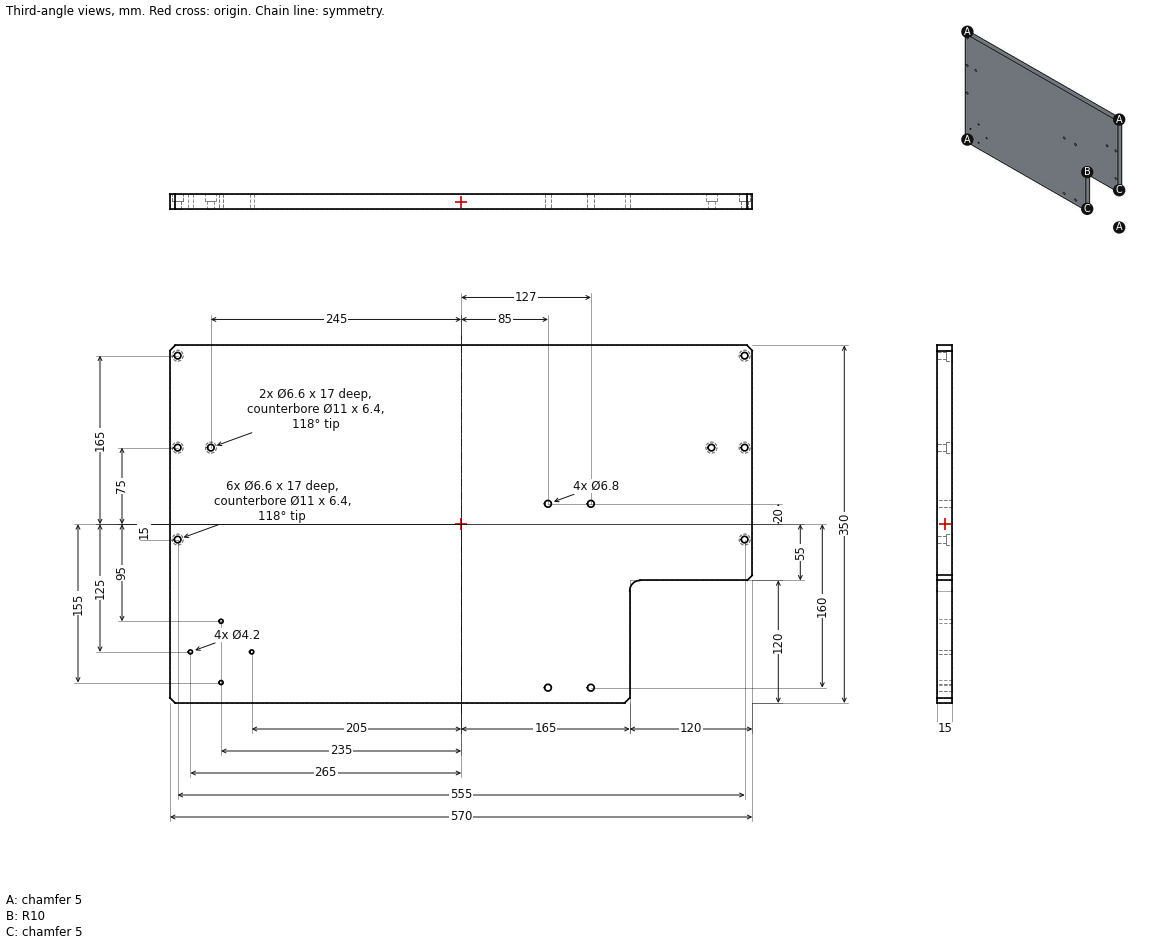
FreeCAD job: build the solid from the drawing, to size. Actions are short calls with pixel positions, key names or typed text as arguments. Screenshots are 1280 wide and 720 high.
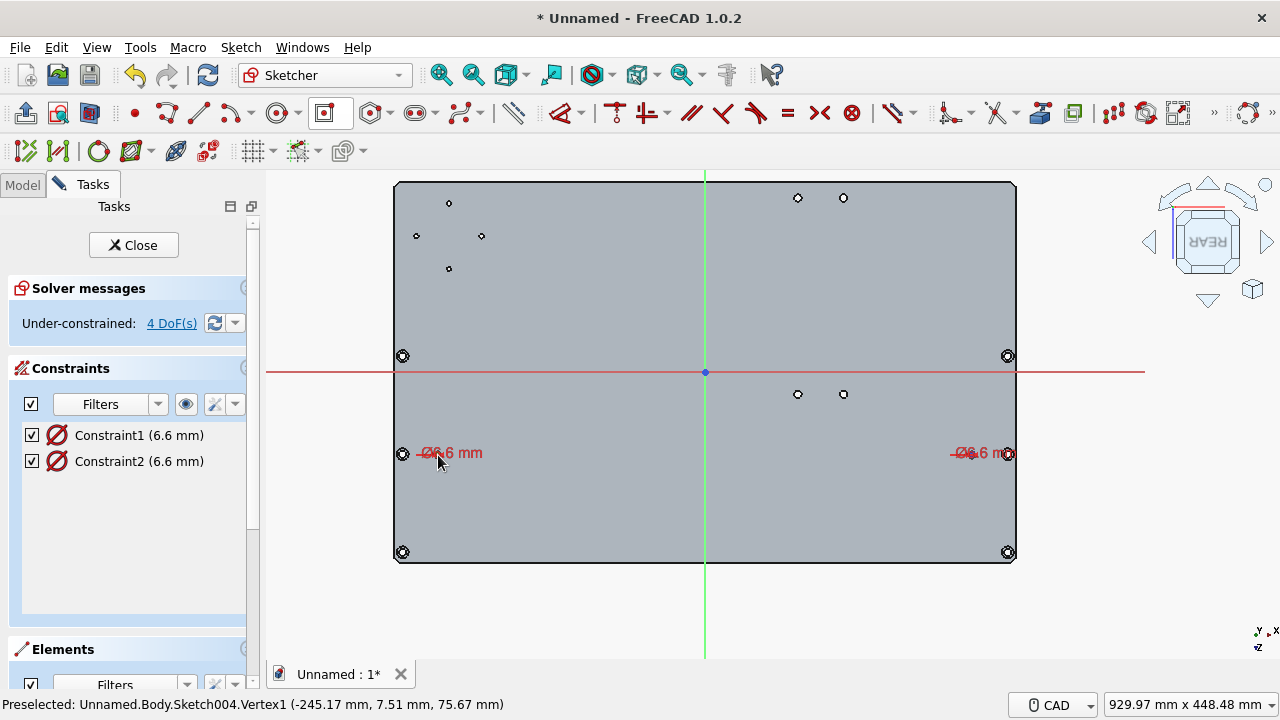
click(972, 455)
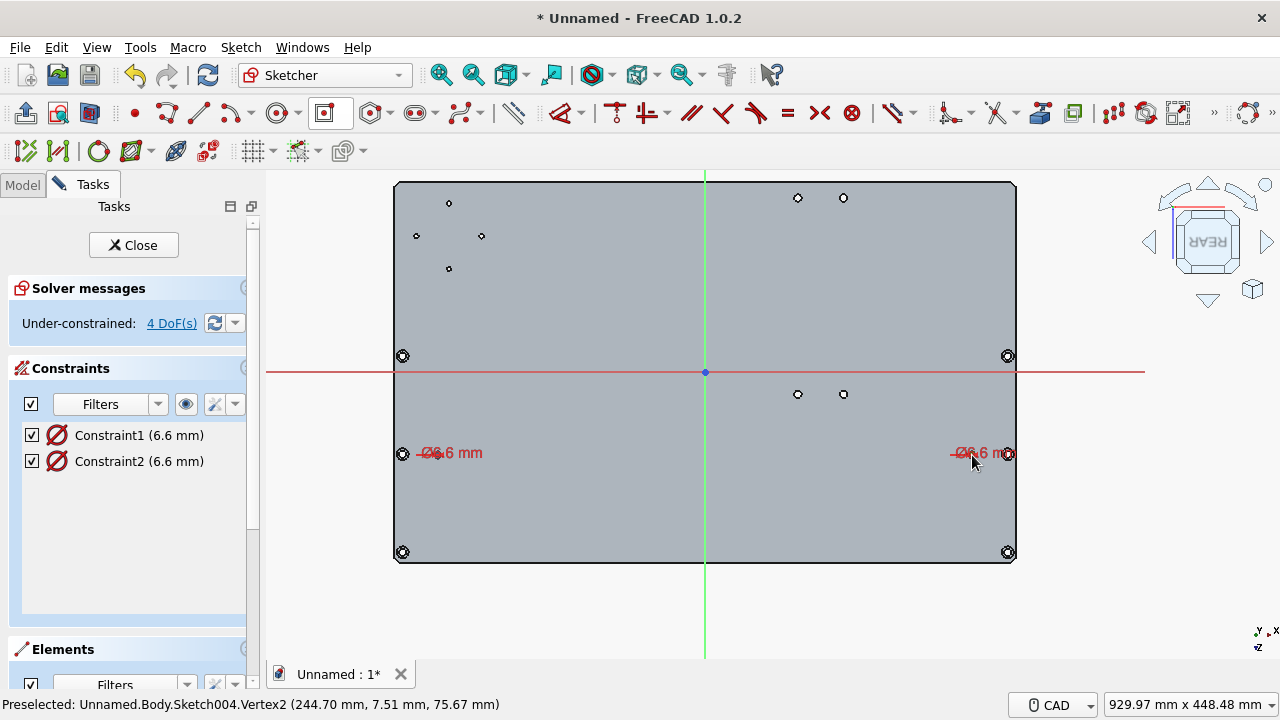
click(705, 600)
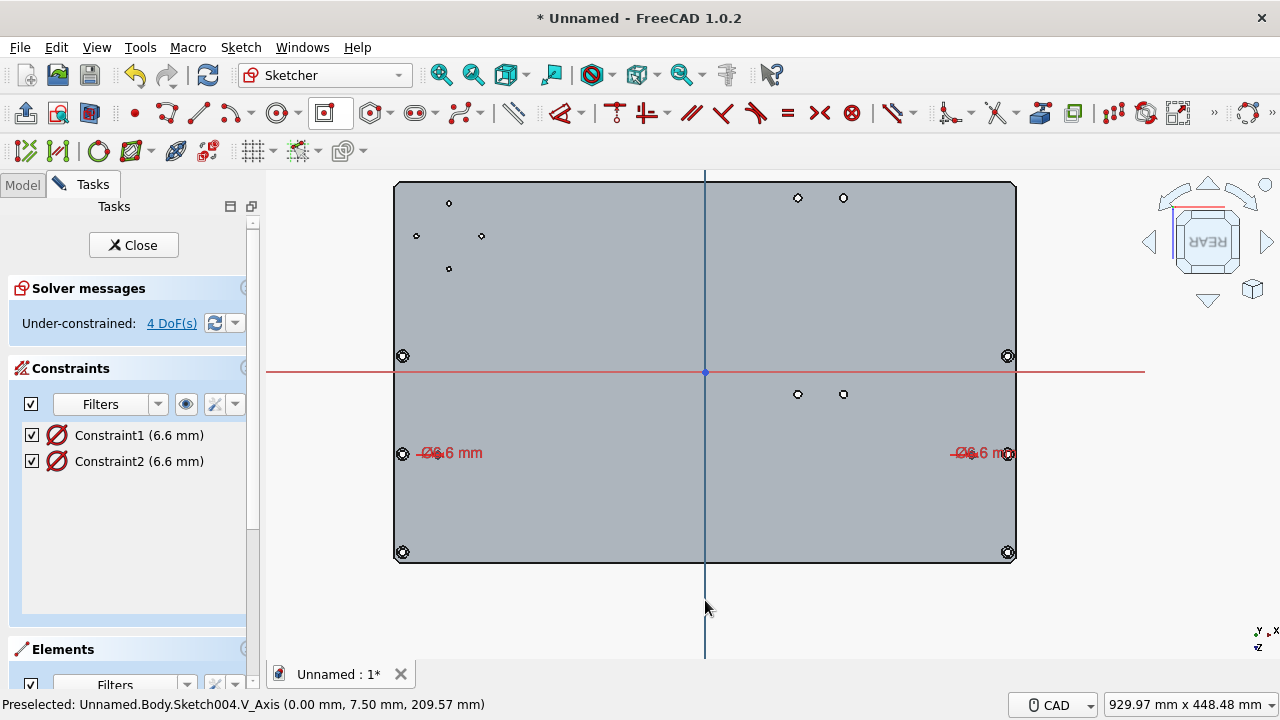
click(820, 114)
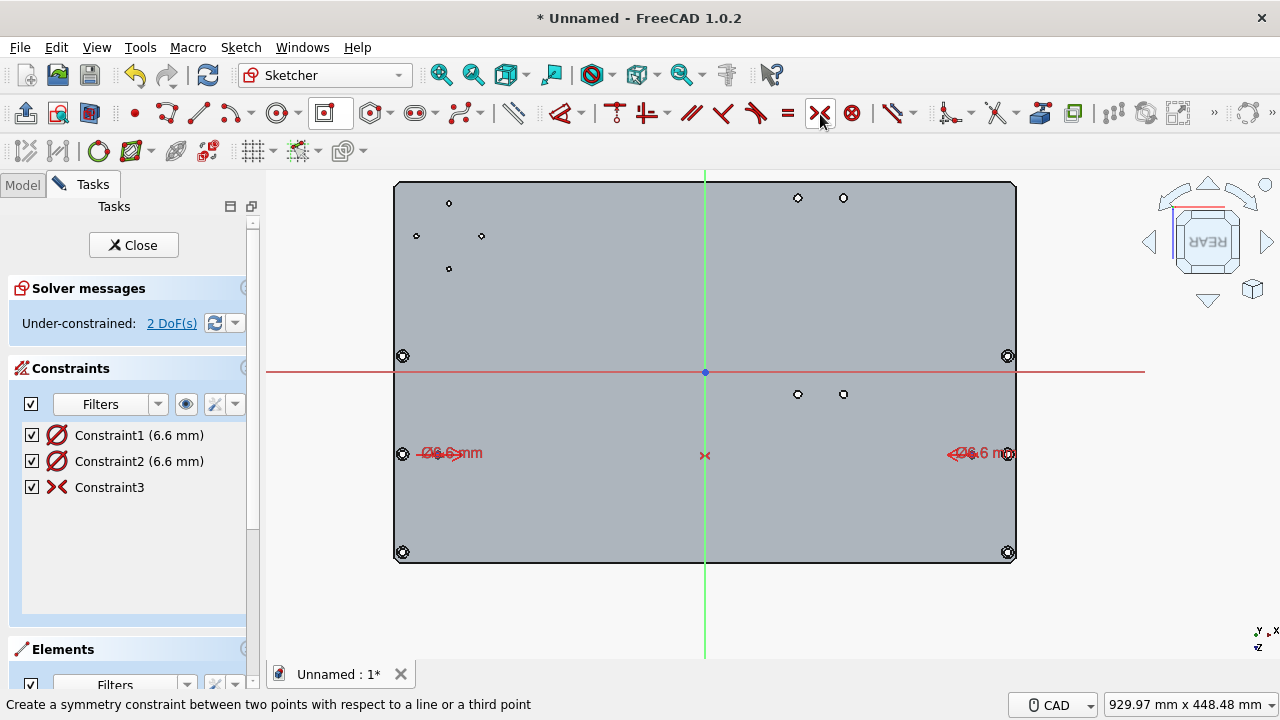
click(560, 114)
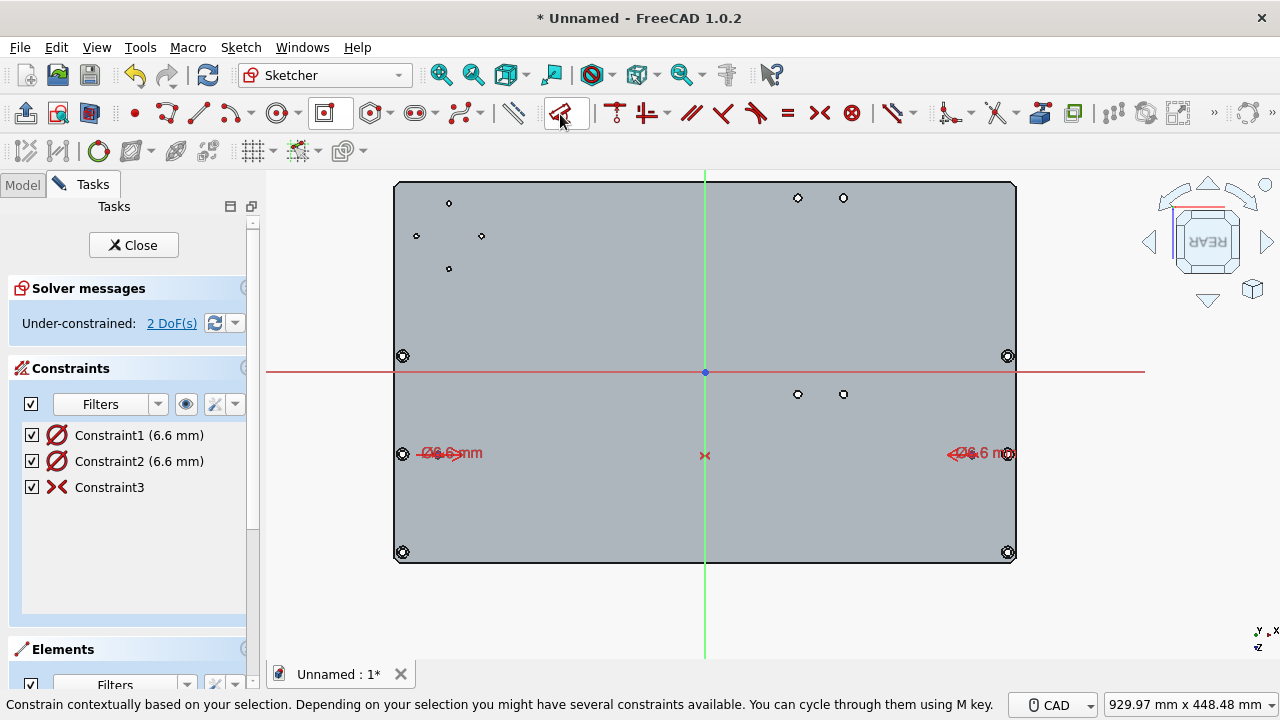
click(438, 455)
click(404, 414)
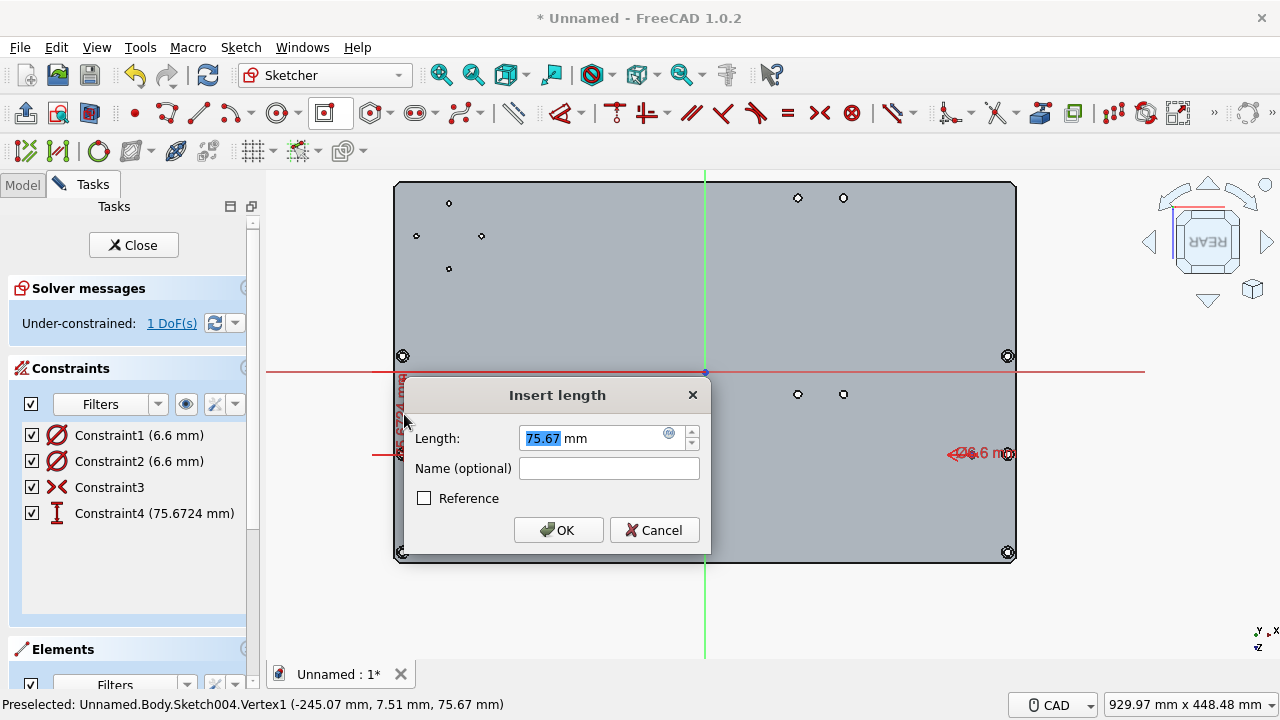
text(75)
key(Return)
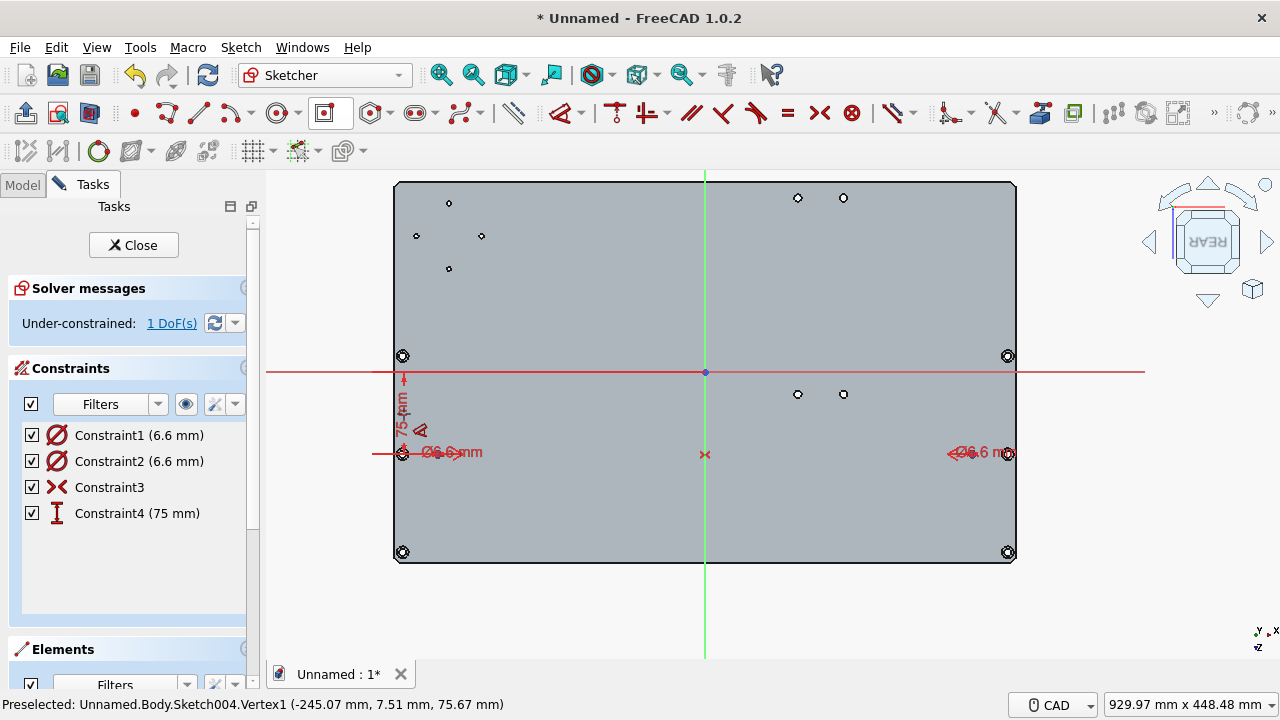
click(438, 454)
click(572, 338)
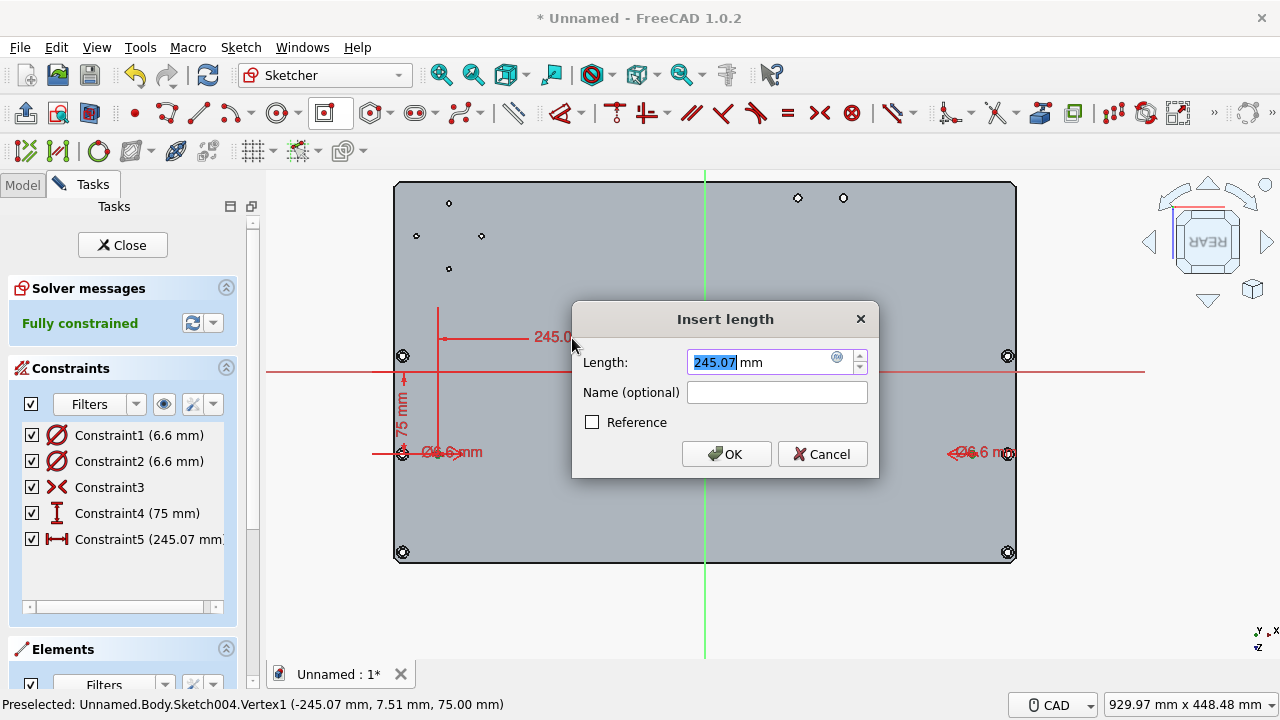
text(245)
key(Return)
key(Escape)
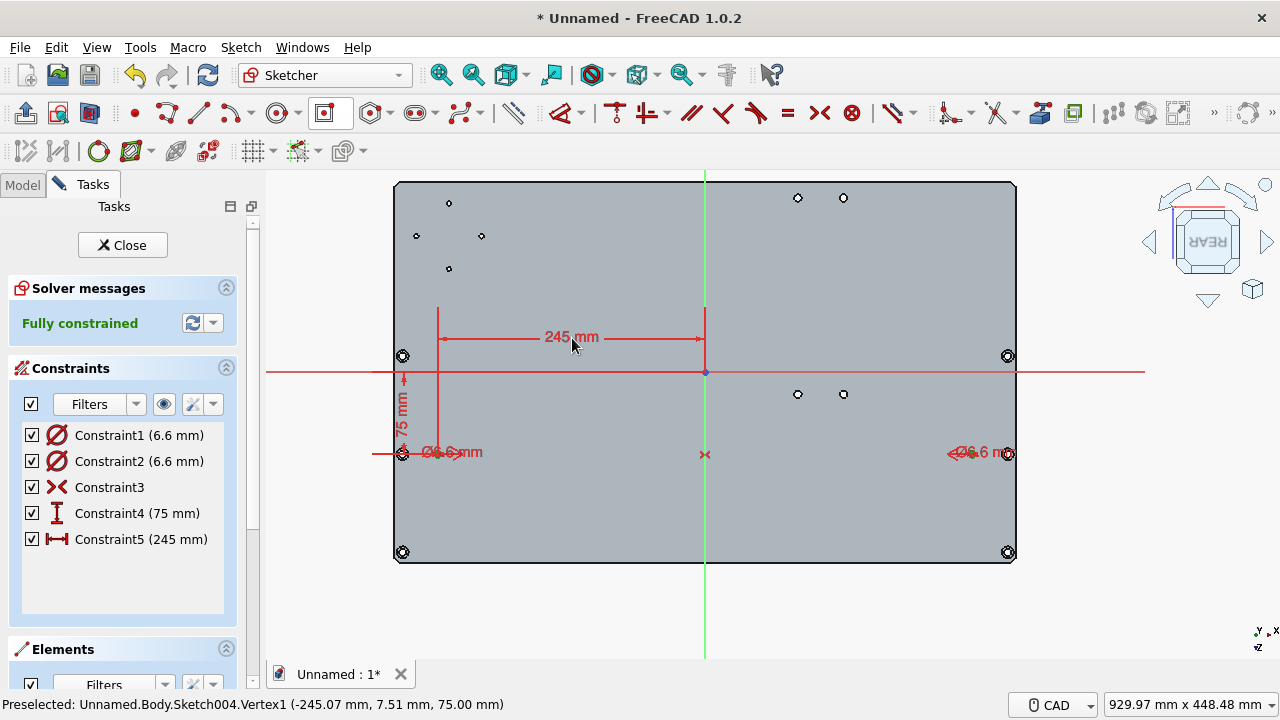
click(123, 245)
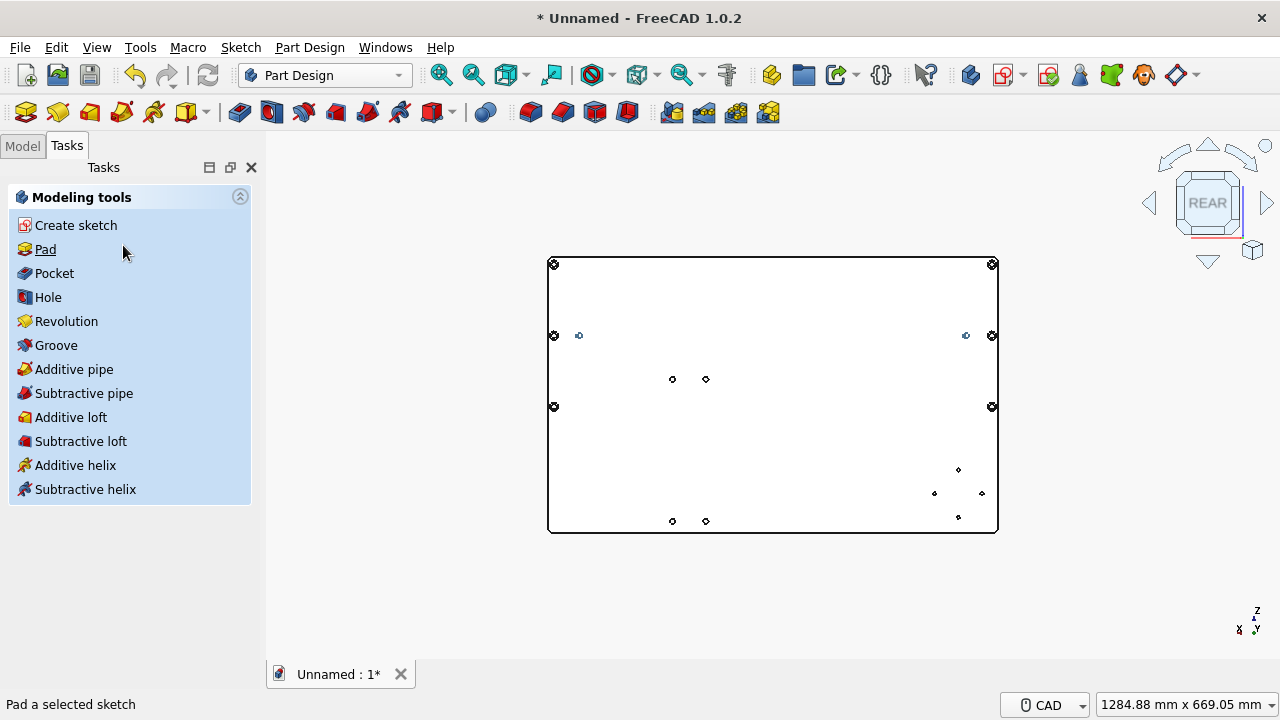
click(272, 112)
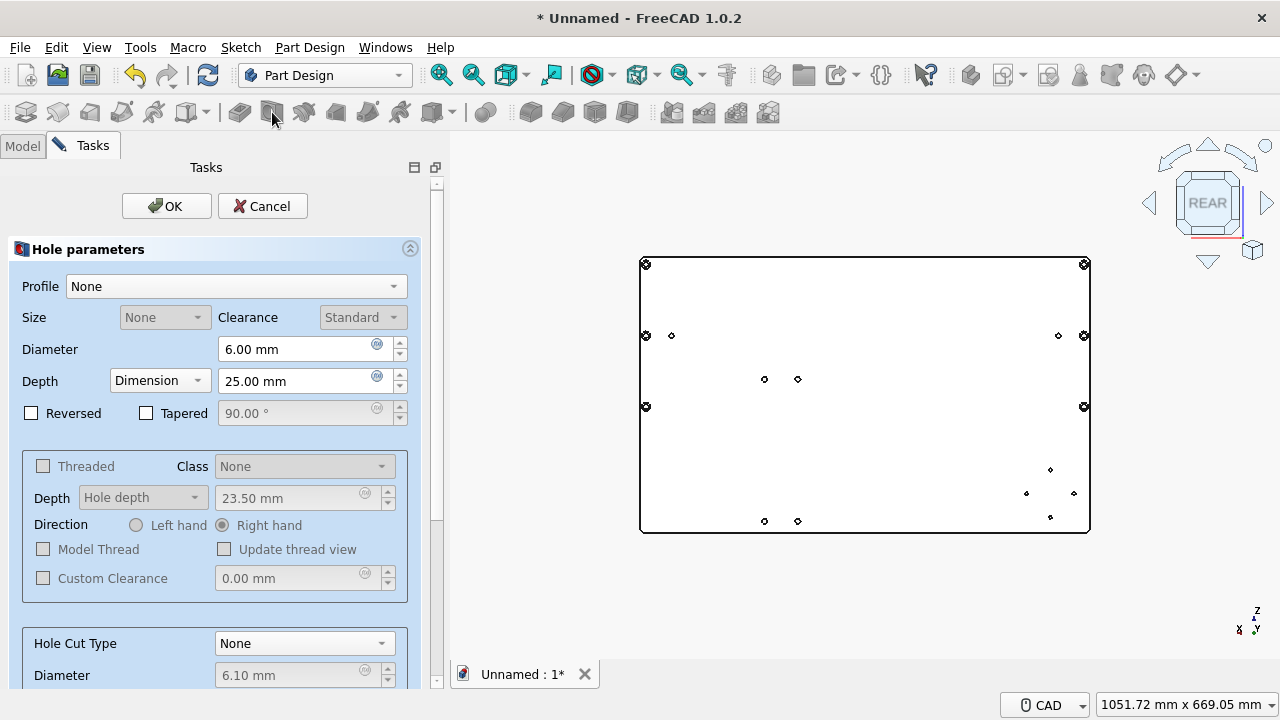
triple_click(305, 349)